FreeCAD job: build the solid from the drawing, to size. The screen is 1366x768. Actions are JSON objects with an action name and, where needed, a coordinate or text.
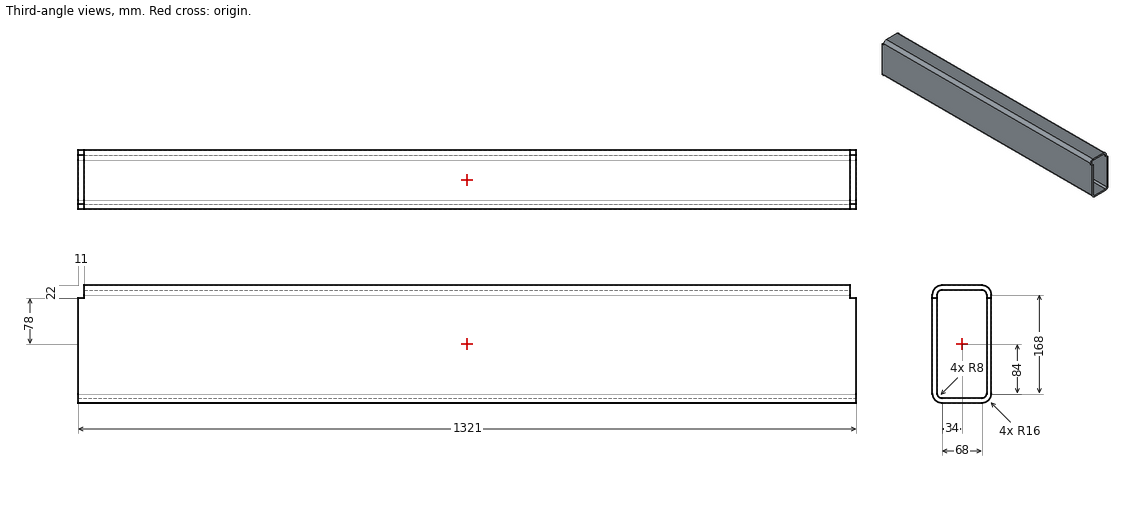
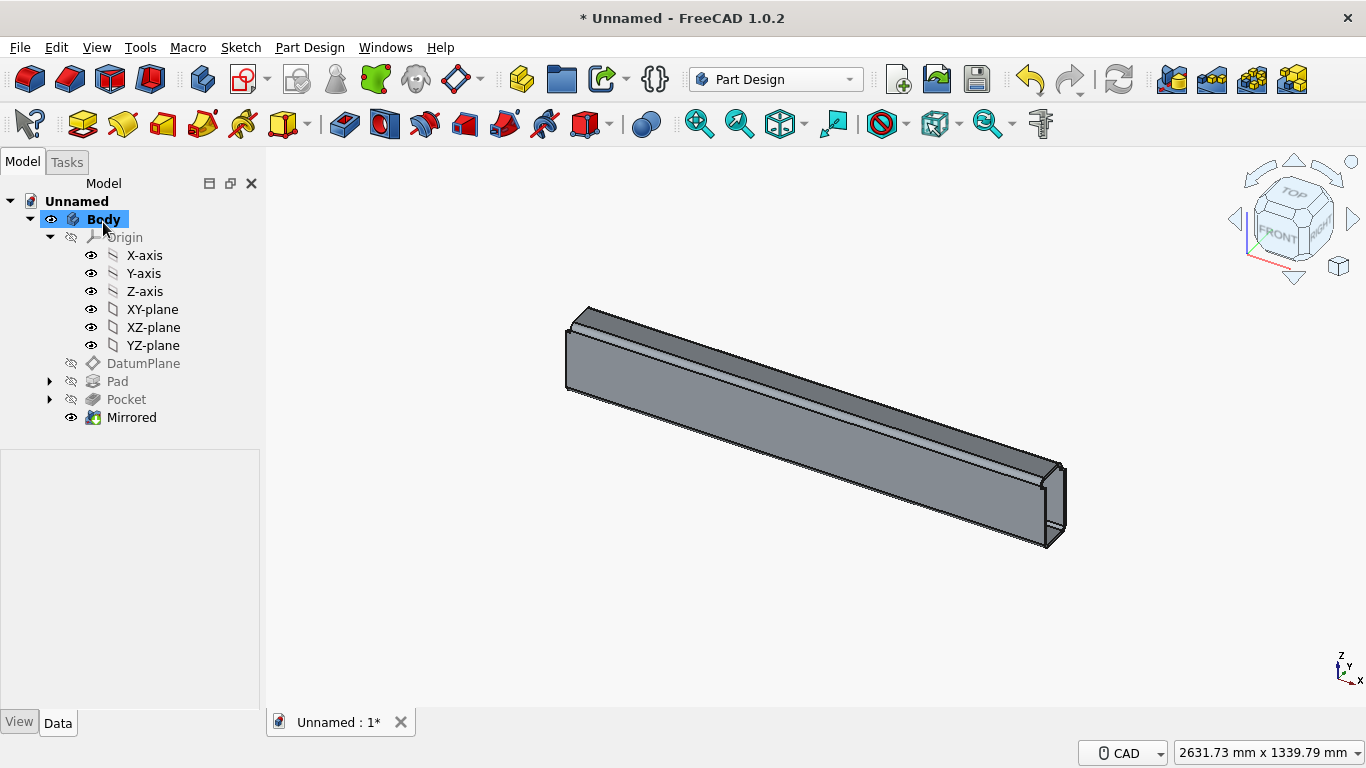
{"action": "key", "text": "0"}